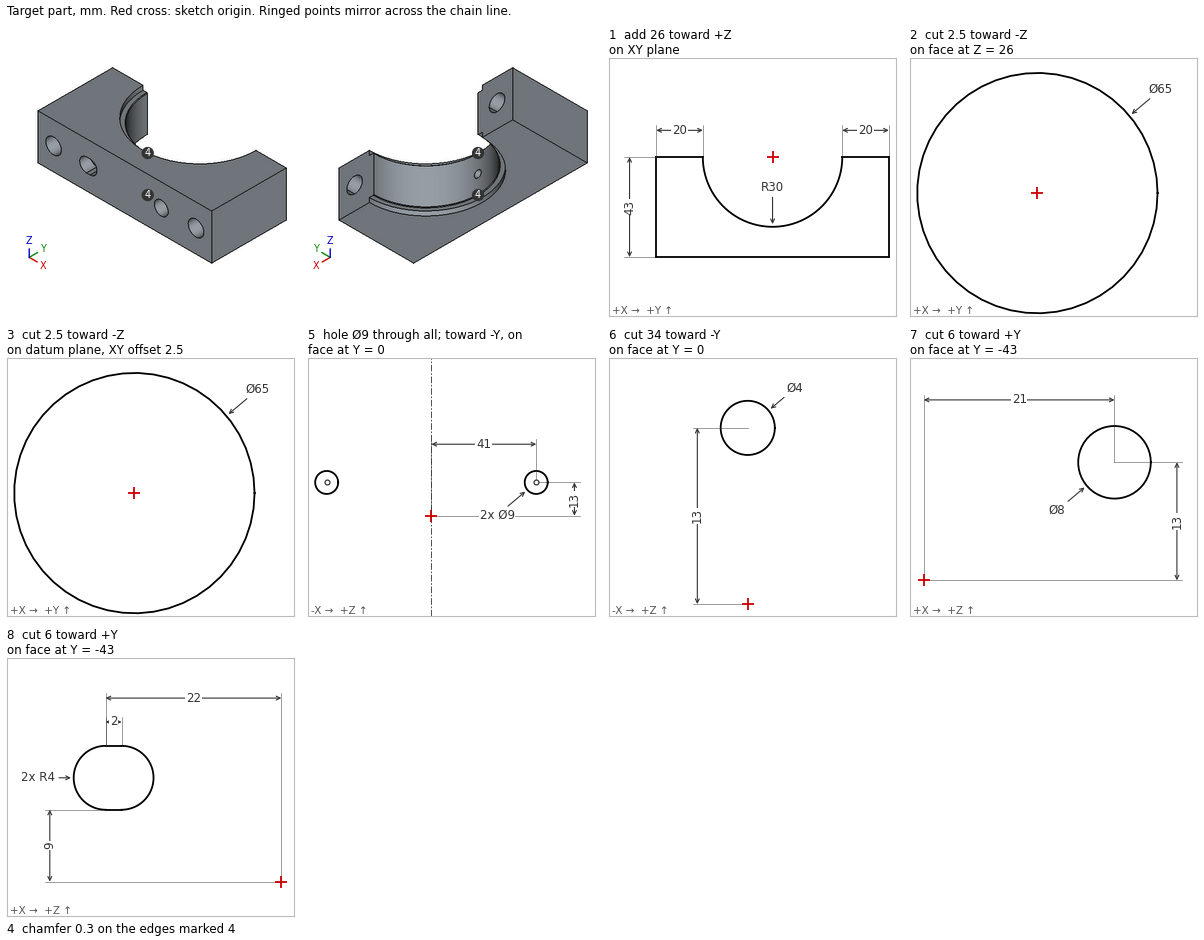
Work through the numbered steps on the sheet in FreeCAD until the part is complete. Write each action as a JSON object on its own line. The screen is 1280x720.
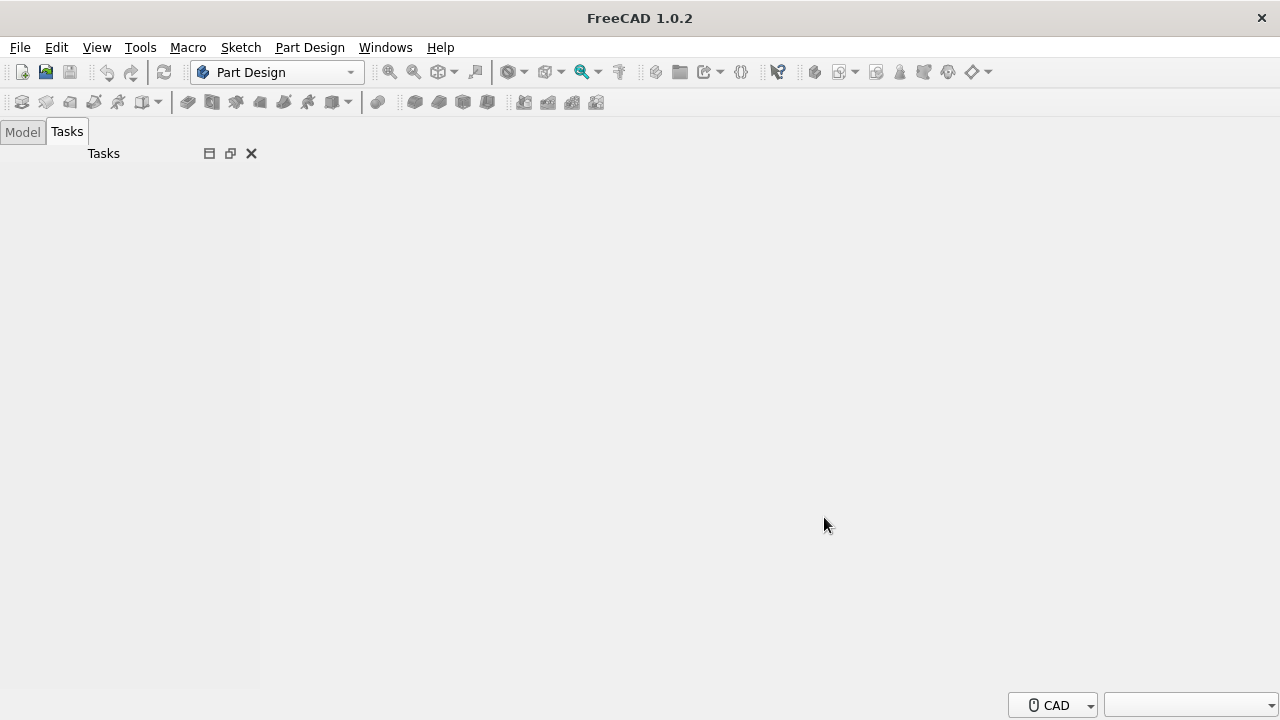
{"action": "left_click", "coordinate": [22, 72]}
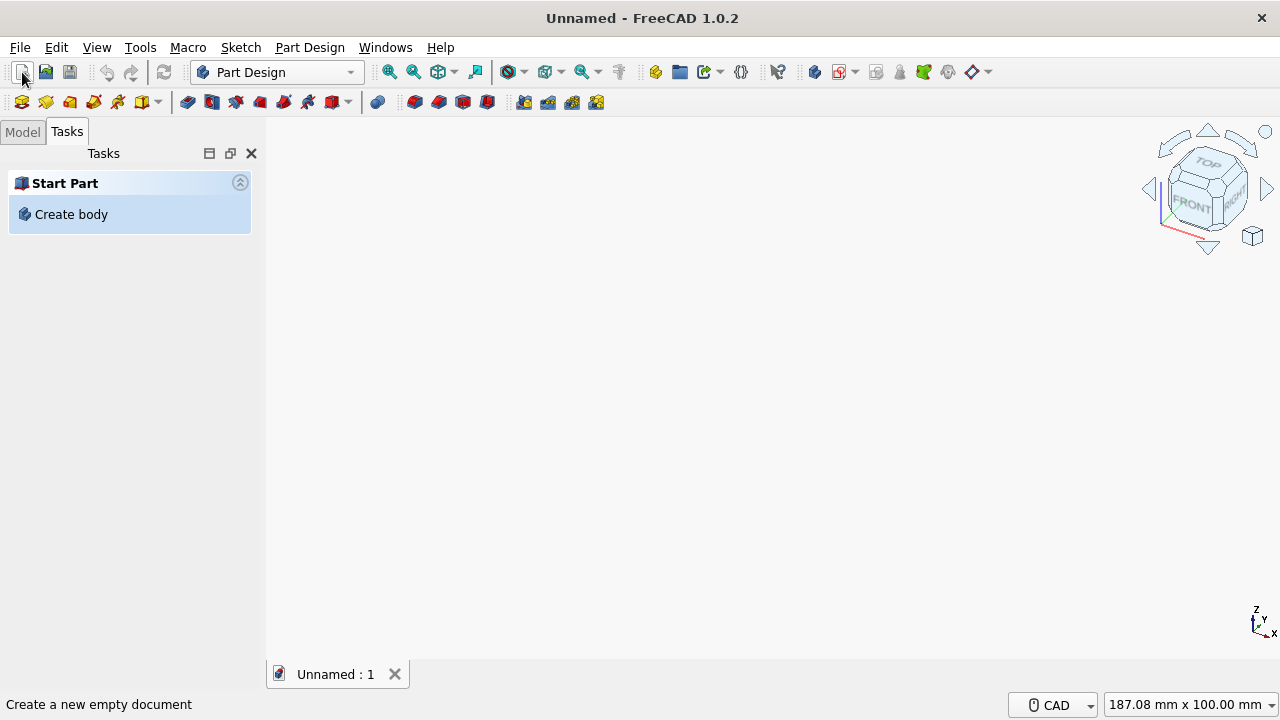
{"action": "left_click", "coordinate": [840, 72]}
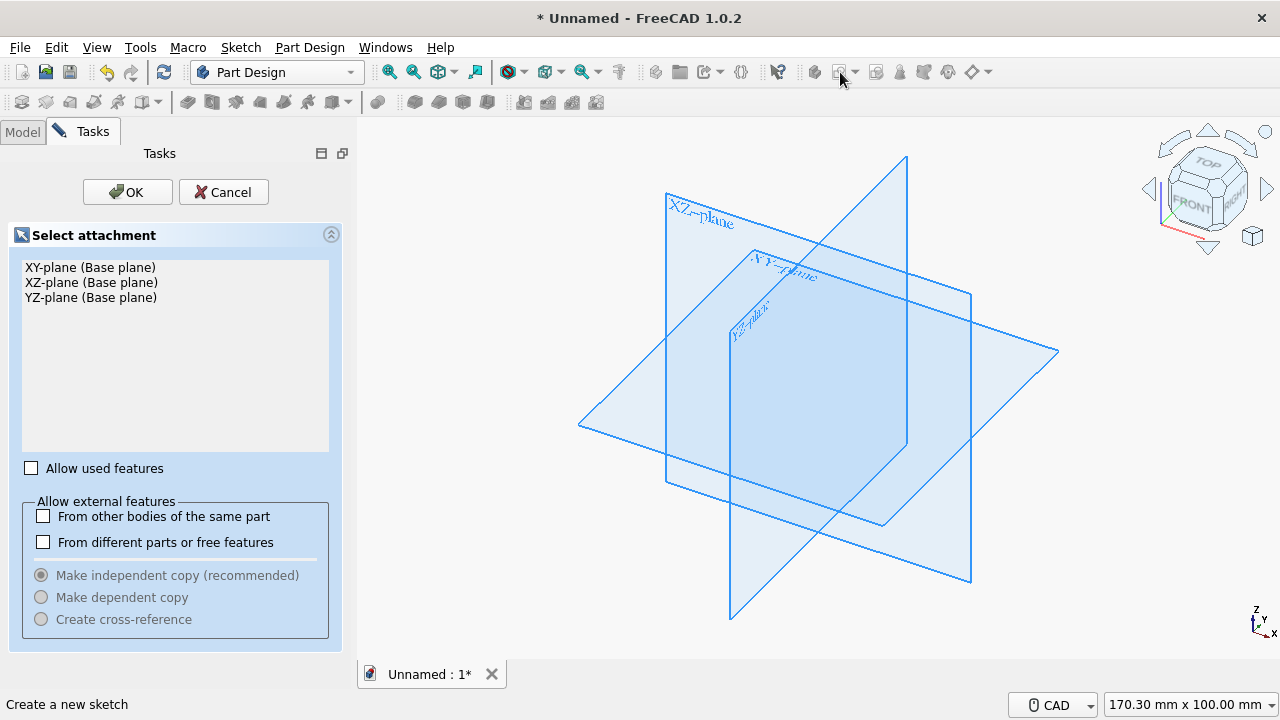
{"action": "left_click", "coordinate": [82, 268]}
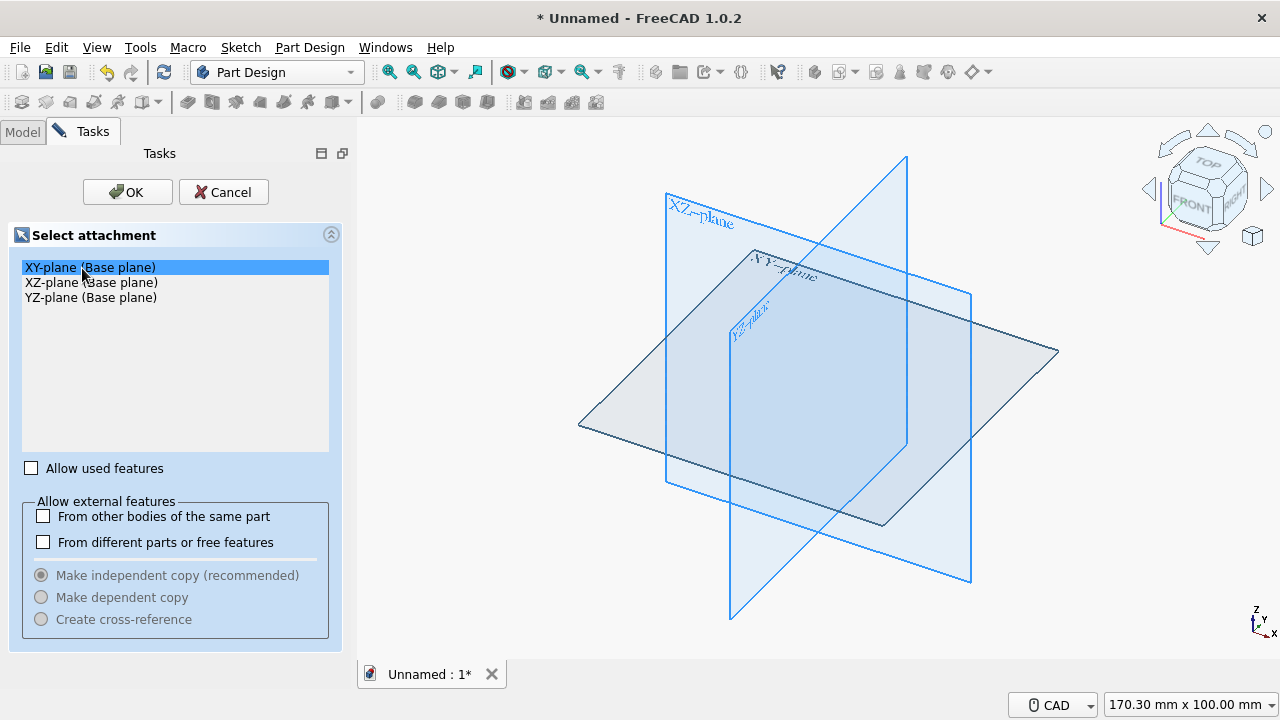
{"action": "left_click", "coordinate": [128, 192]}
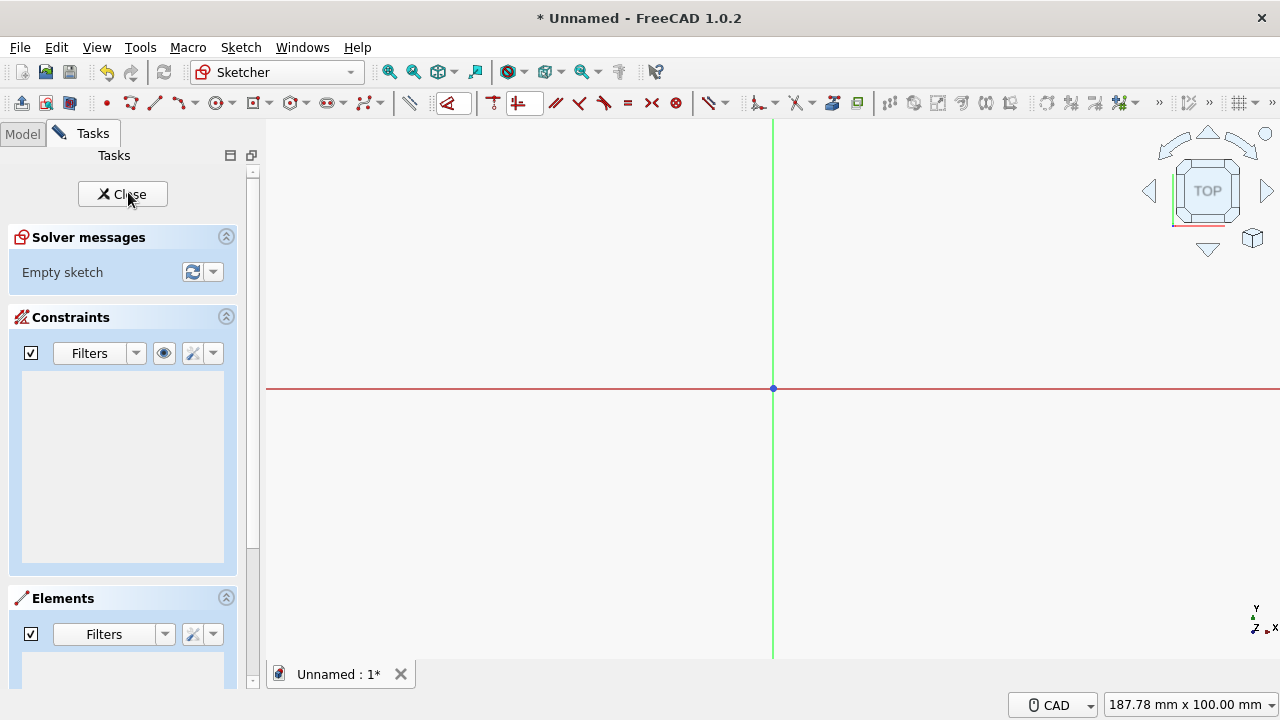
{"action": "scroll", "coordinate": [395, 147], "scroll_direction": "down", "scroll_amount": 1}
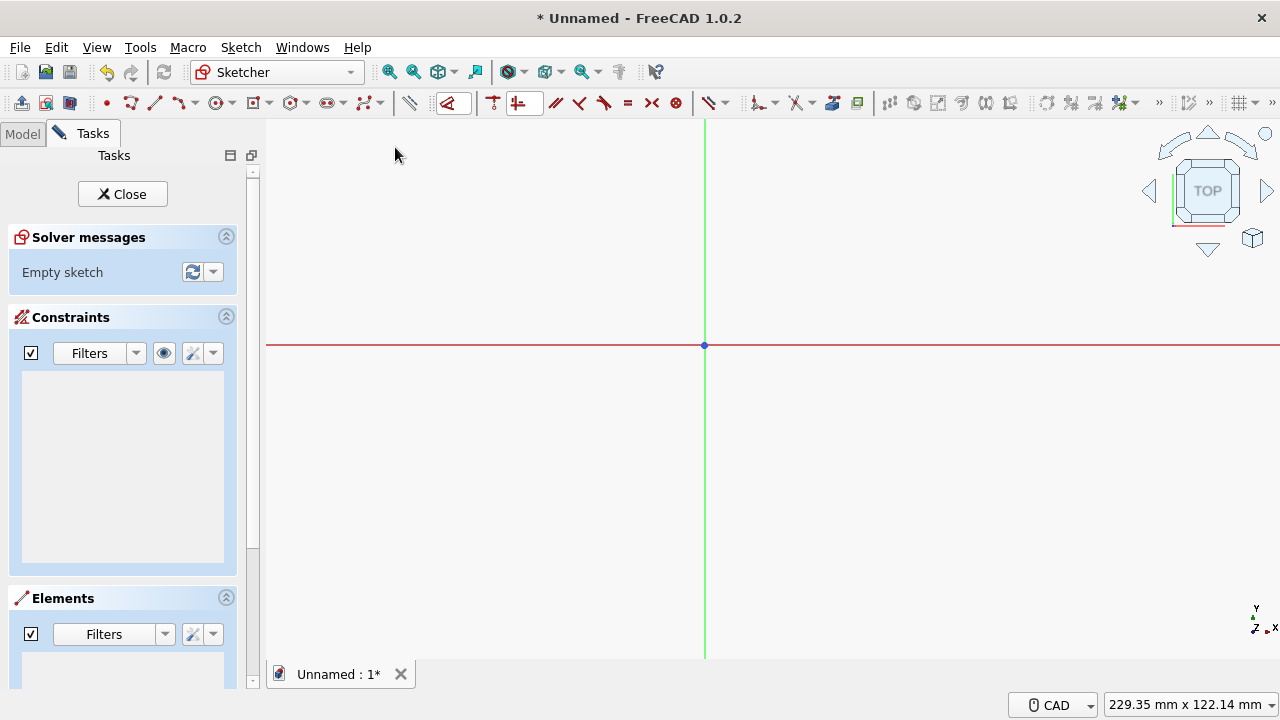
{"action": "left_click", "coordinate": [132, 104]}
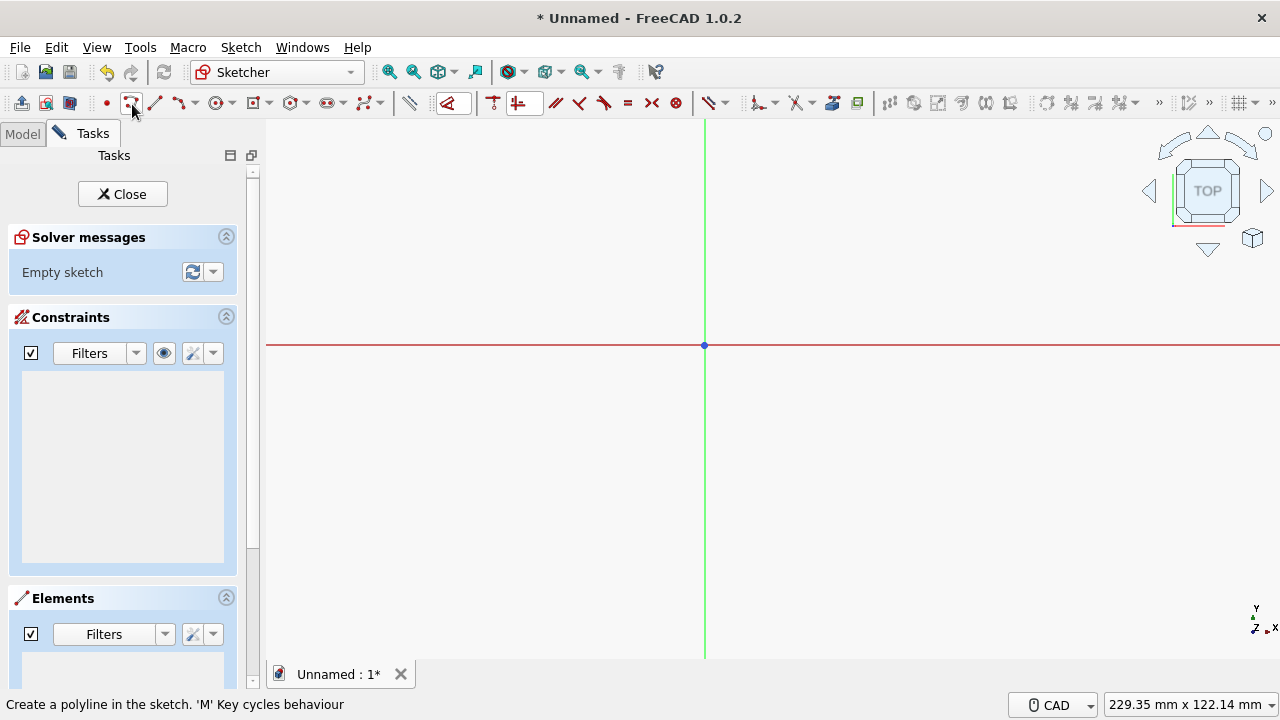
{"action": "left_click", "coordinate": [572, 345]}
{"action": "left_click", "coordinate": [483, 354]}
{"action": "left_click", "coordinate": [483, 535]}
{"action": "left_click", "coordinate": [926, 535]}
{"action": "left_click", "coordinate": [926, 345]}
{"action": "left_click", "coordinate": [837, 354]}
{"action": "right_click", "coordinate": [837, 354]}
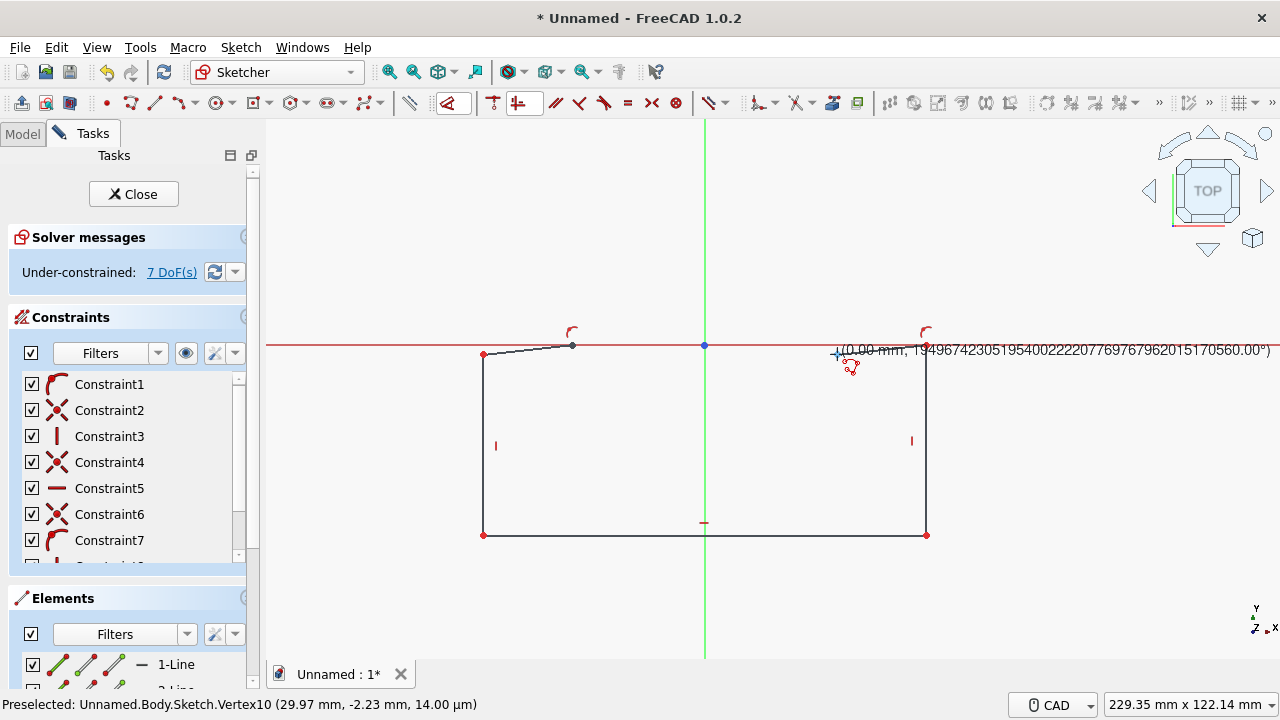
{"action": "left_click", "coordinate": [180, 104]}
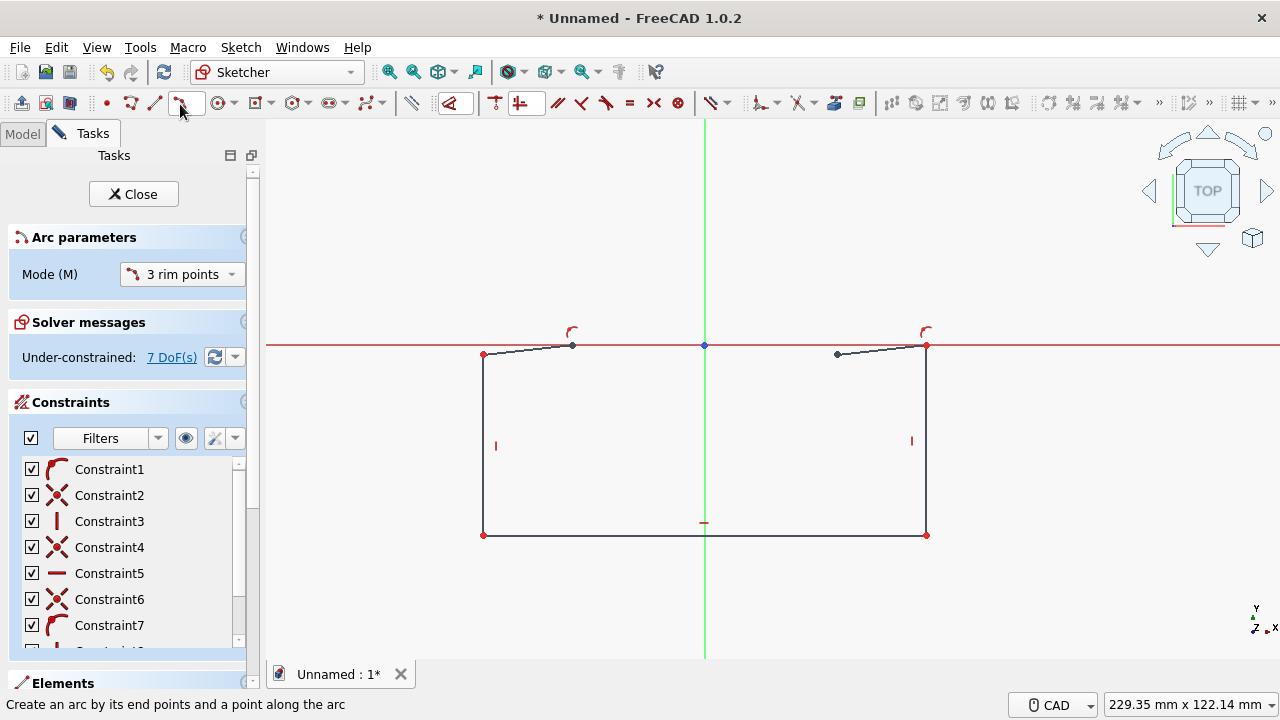
{"action": "left_click", "coordinate": [837, 355]}
{"action": "left_click", "coordinate": [572, 345]}
{"action": "left_click", "coordinate": [664, 471]}
{"action": "key", "text": "Escape"}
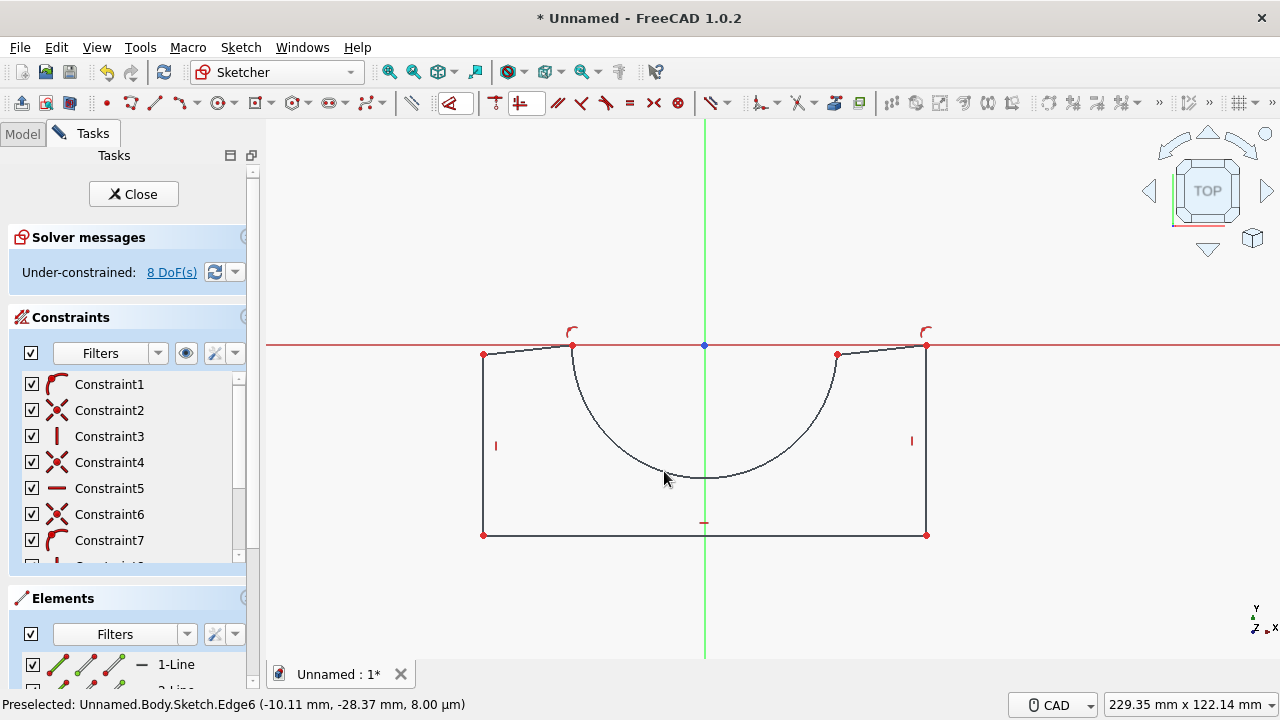
{"action": "left_click", "coordinate": [545, 348]}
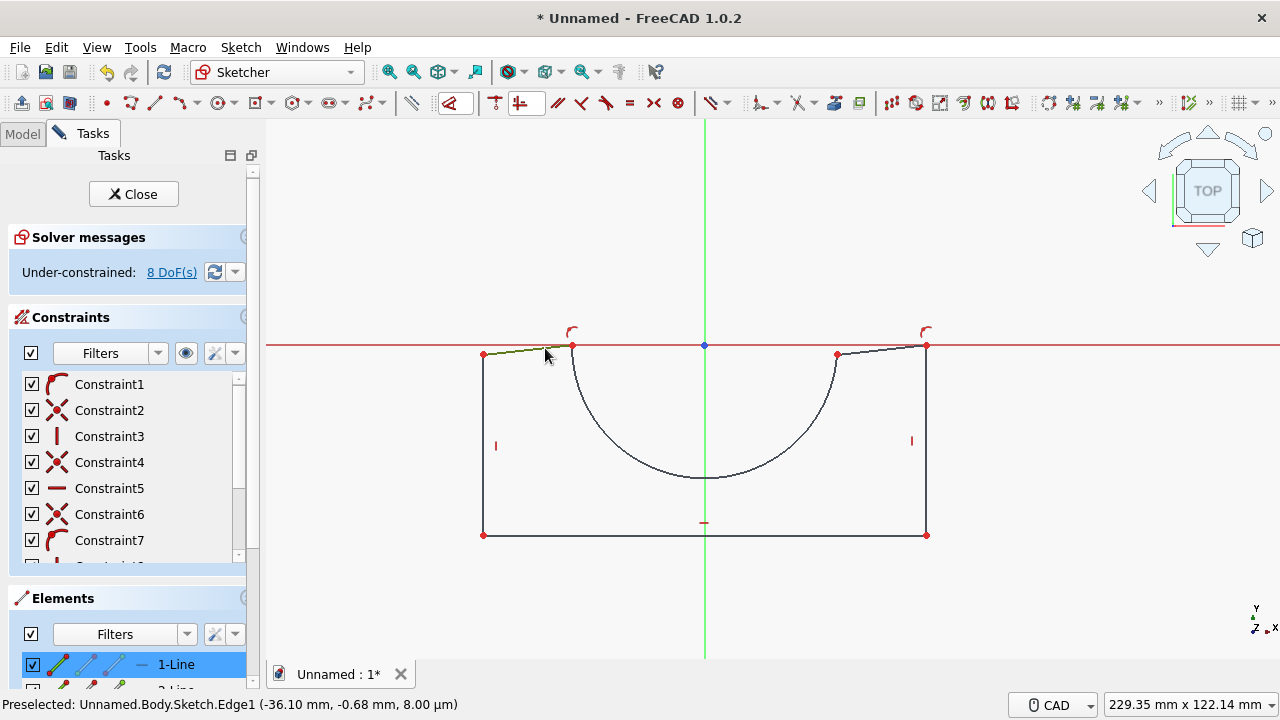
{"action": "left_click", "coordinate": [540, 104]}